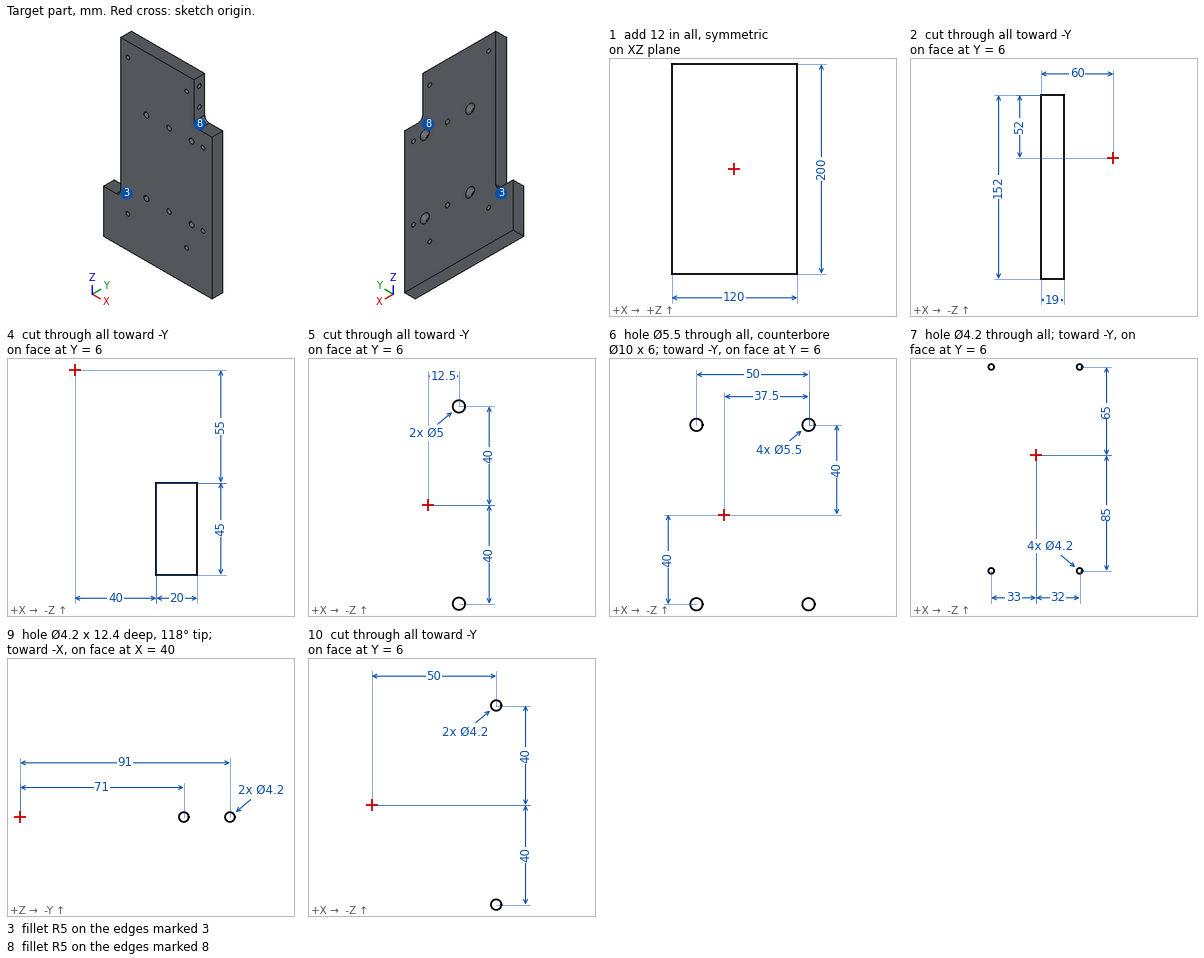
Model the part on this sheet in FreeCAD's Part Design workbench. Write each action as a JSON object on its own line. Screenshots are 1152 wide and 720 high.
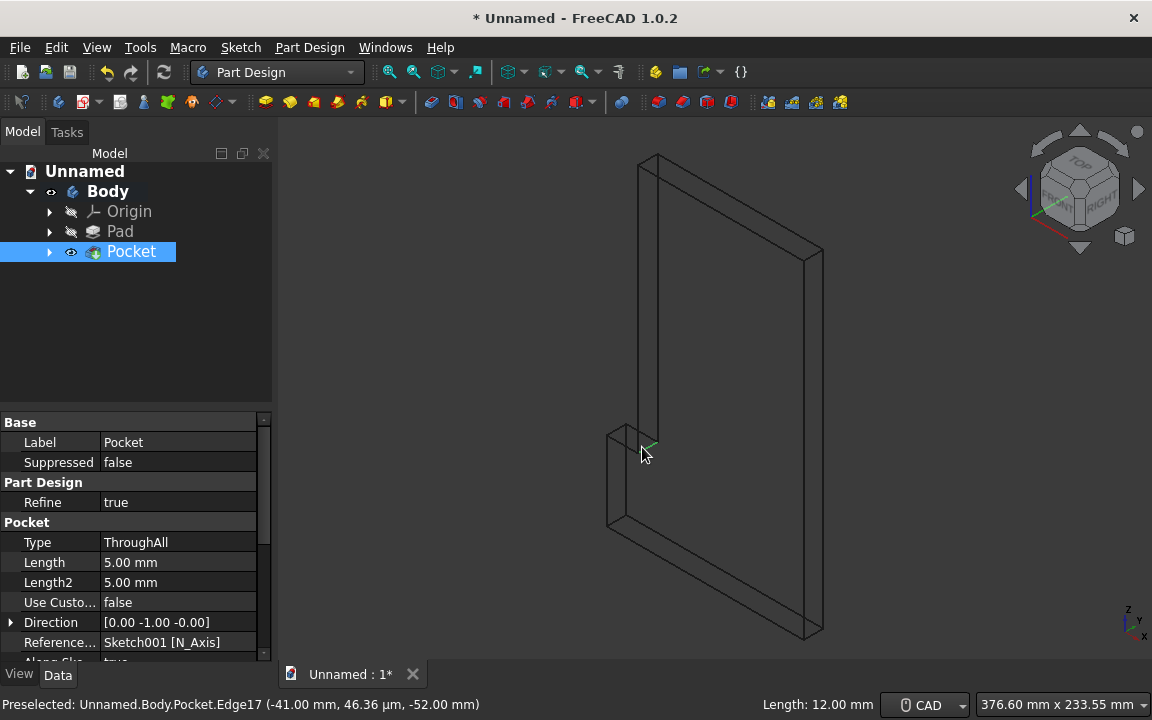
{"action": "key", "text": "v 1"}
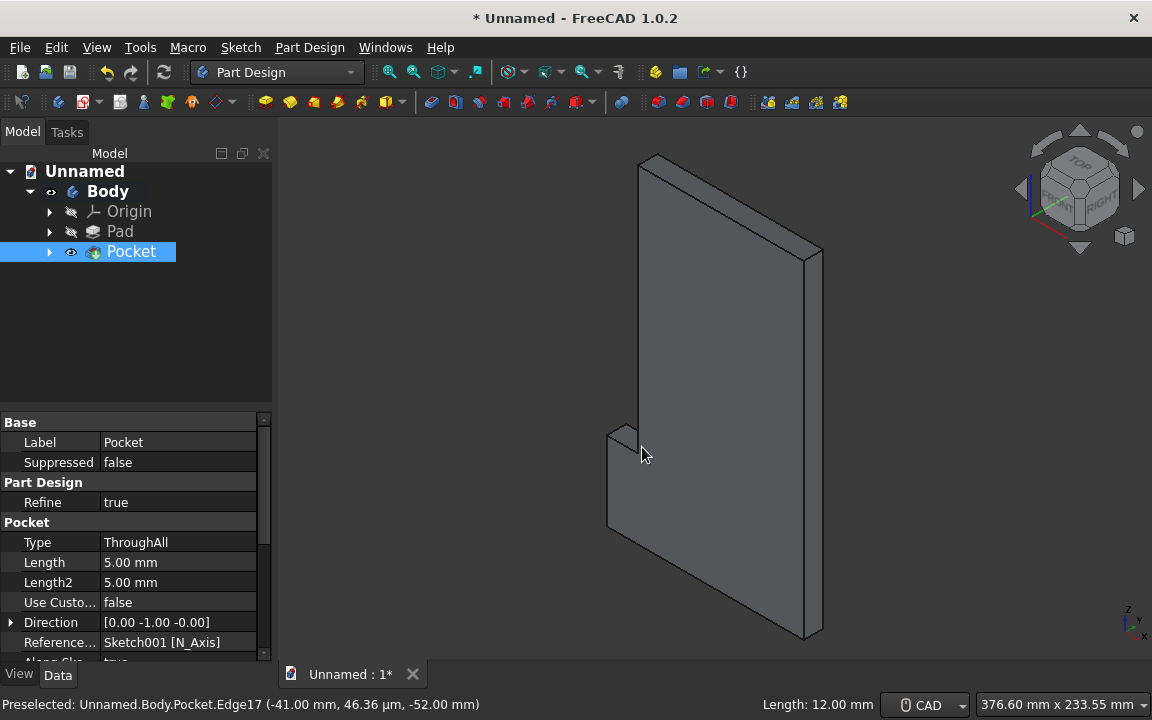
{"action": "left_click", "coordinate": [660, 102]}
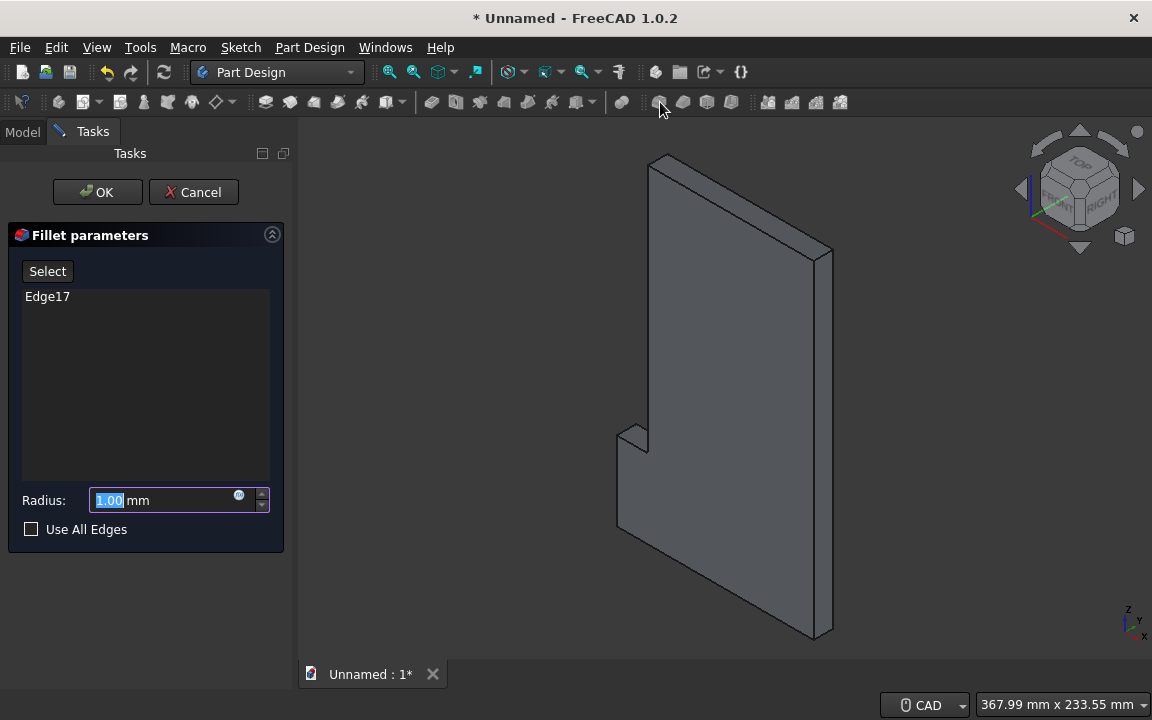
{"action": "type", "text": "5"}
{"action": "key", "text": "Tab"}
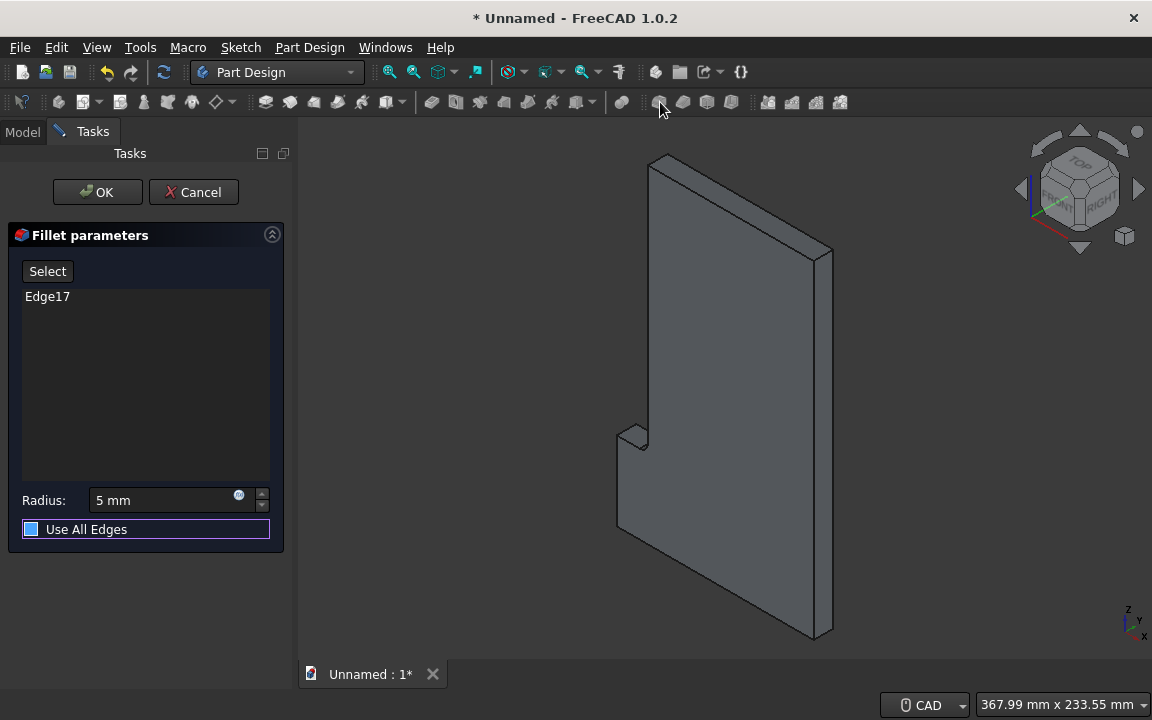
{"action": "left_click", "coordinate": [98, 192]}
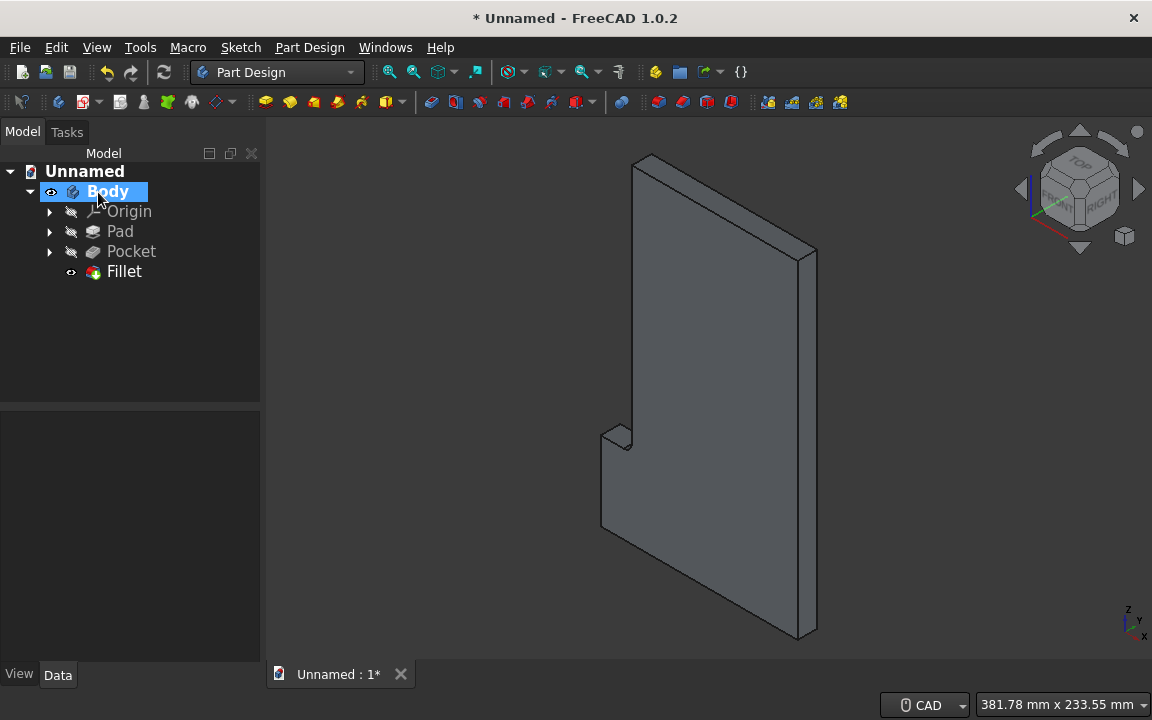
{"action": "key", "text": "4"}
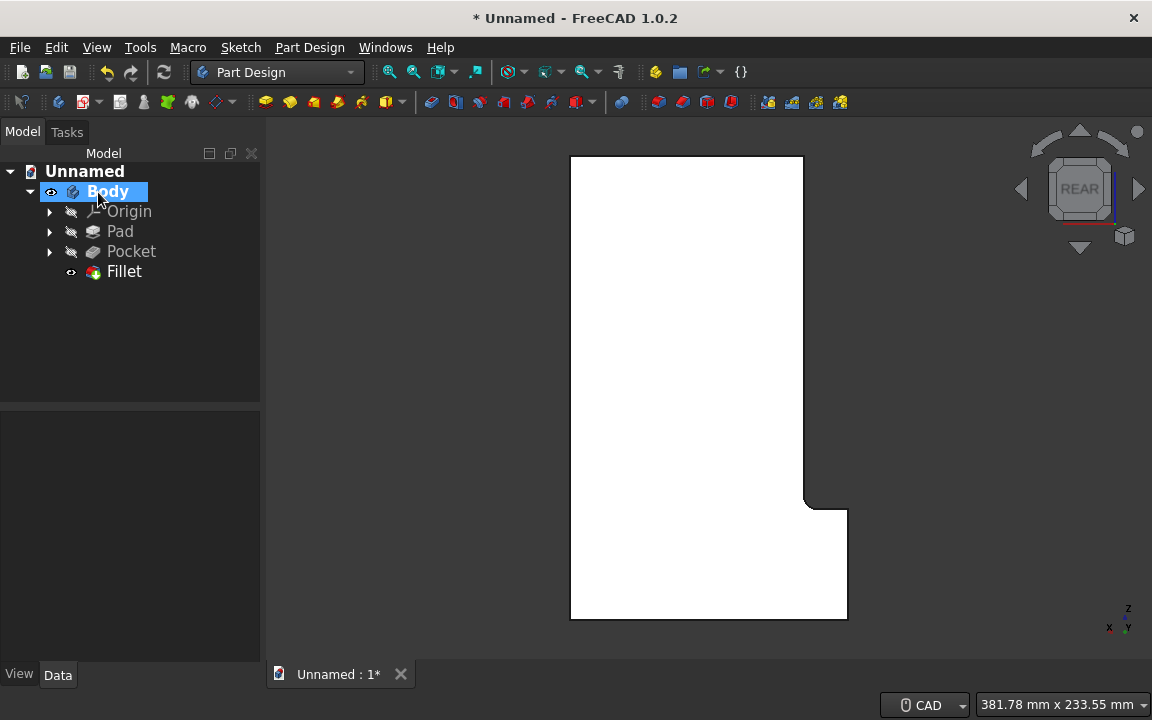
{"action": "left_click", "coordinate": [669, 321]}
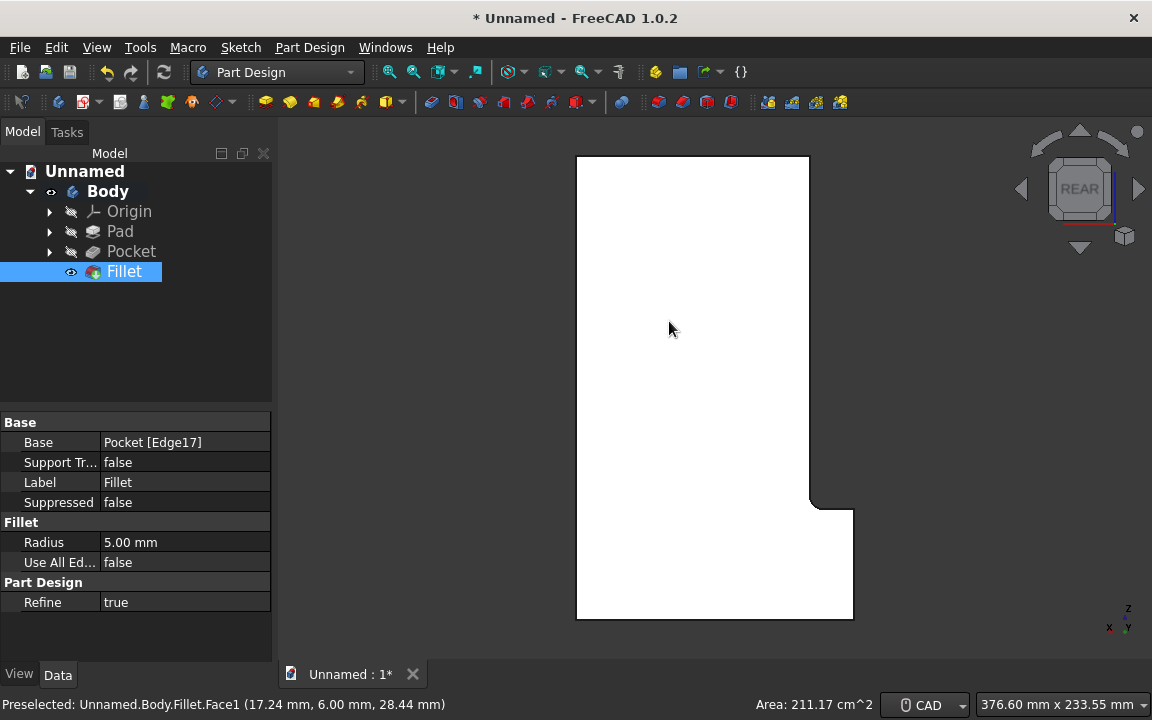
{"action": "left_click", "coordinate": [84, 102]}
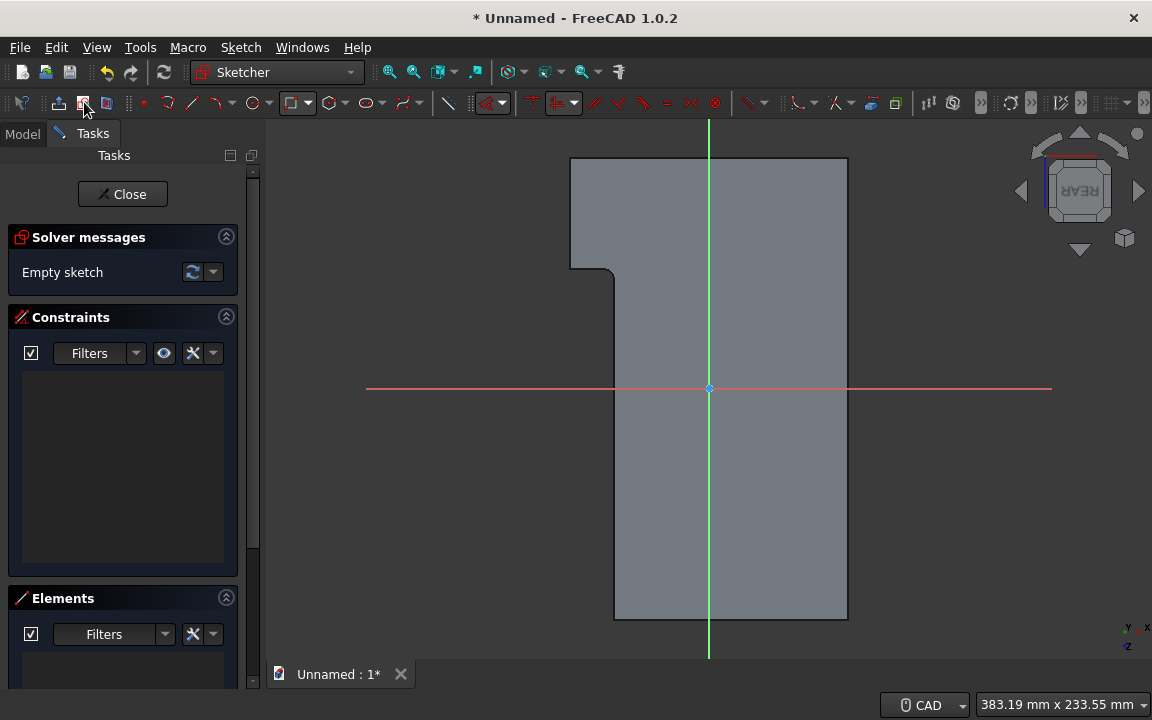
{"action": "scroll", "coordinate": [294, 147], "scroll_direction": "down", "scroll_amount": 1}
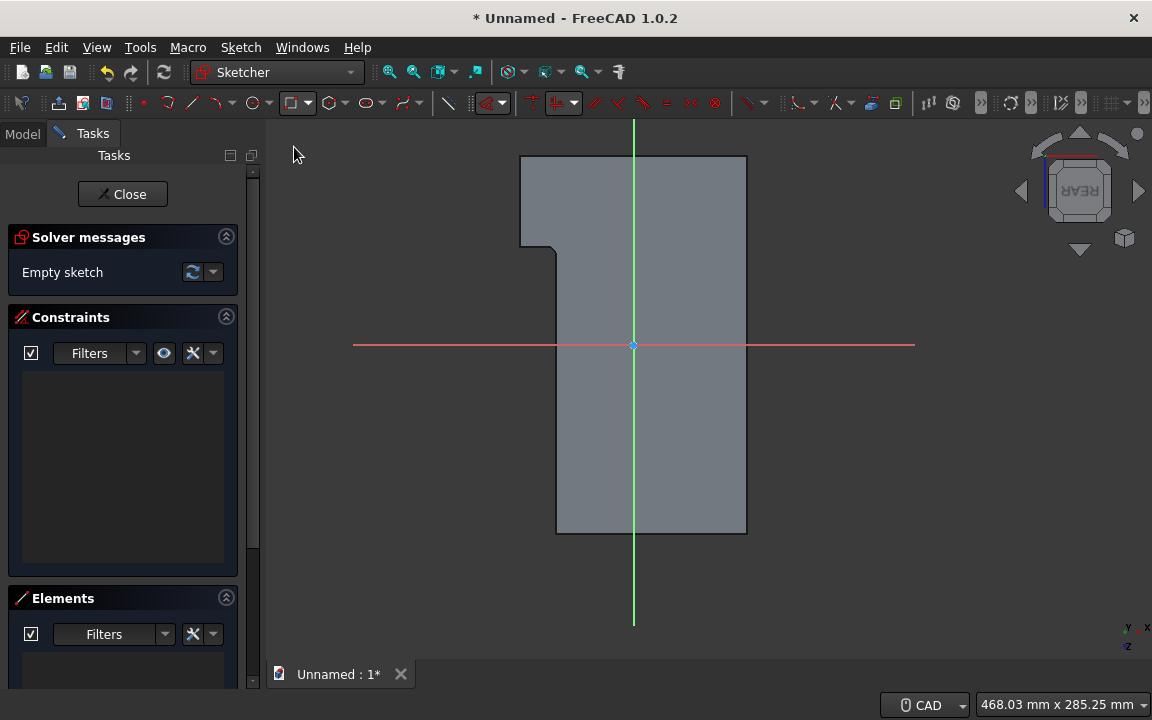
{"action": "scroll", "coordinate": [751, 502], "scroll_direction": "up", "scroll_amount": 3}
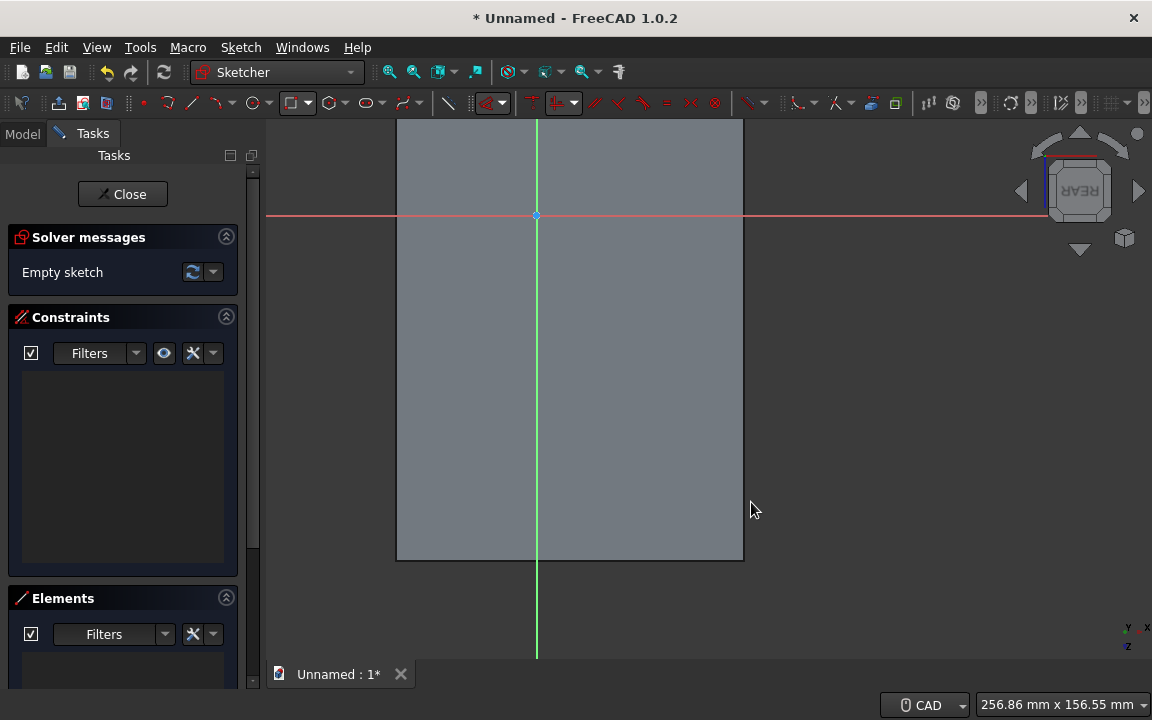
{"action": "left_click", "coordinate": [292, 104]}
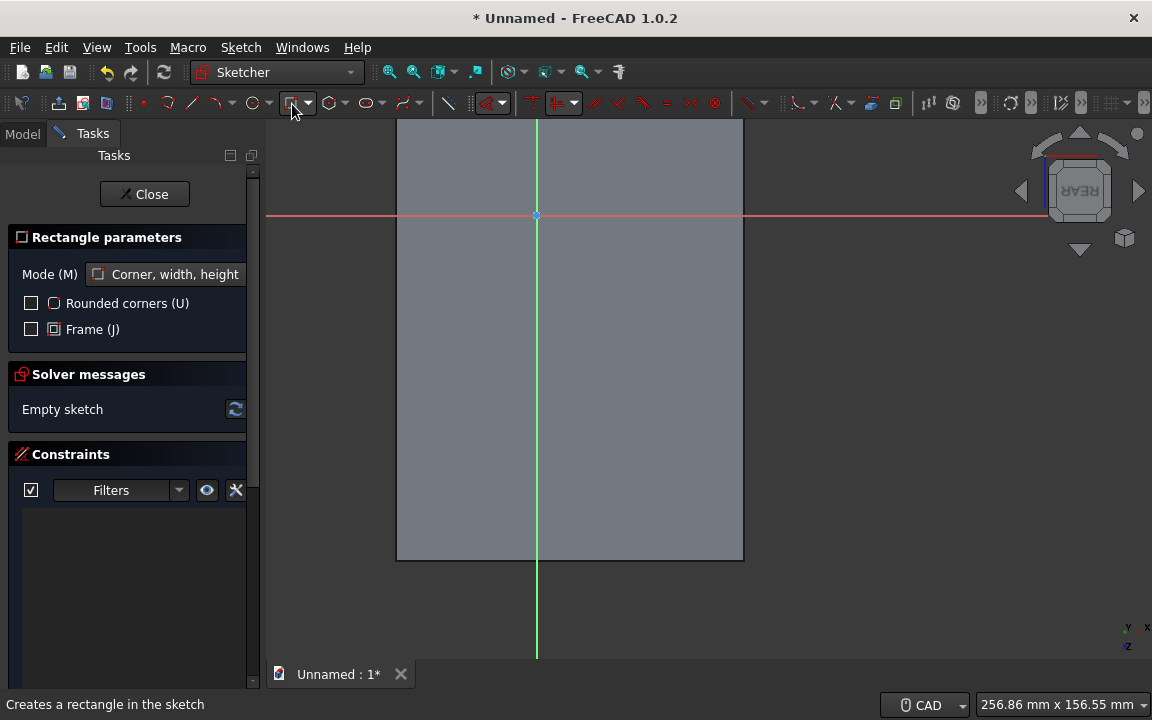
{"action": "left_click", "coordinate": [675, 405]}
{"action": "left_click", "coordinate": [744, 561]}
{"action": "key", "text": "Escape"}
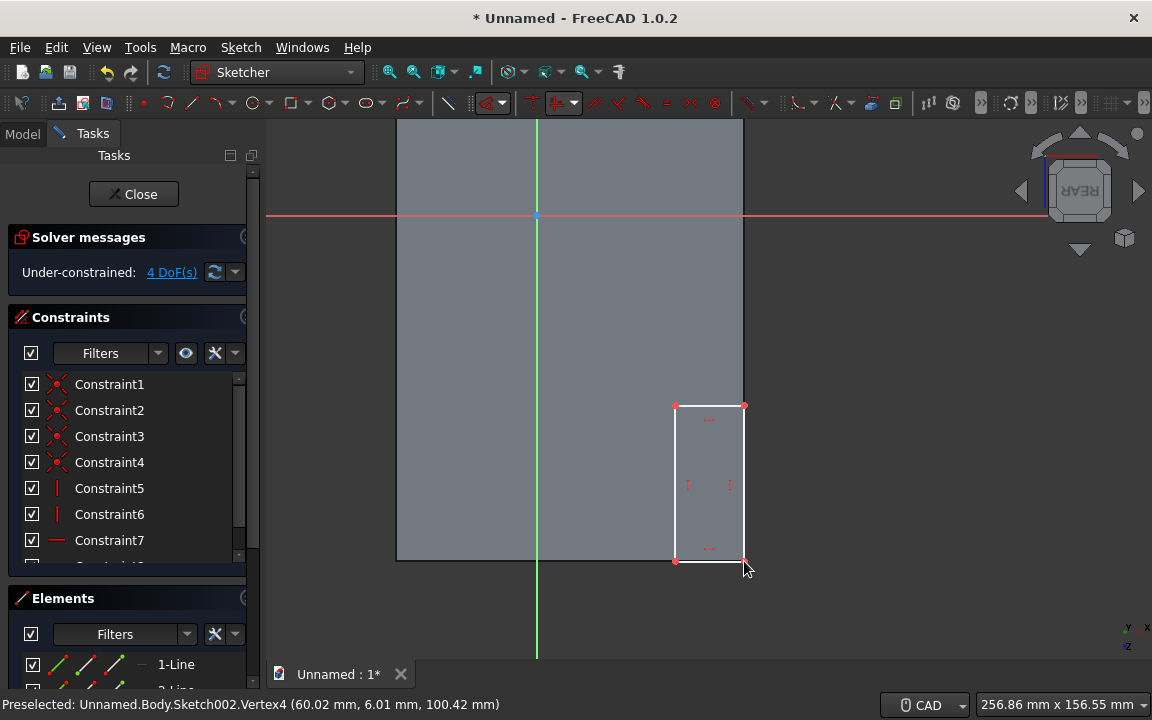
{"action": "left_click", "coordinate": [675, 453]}